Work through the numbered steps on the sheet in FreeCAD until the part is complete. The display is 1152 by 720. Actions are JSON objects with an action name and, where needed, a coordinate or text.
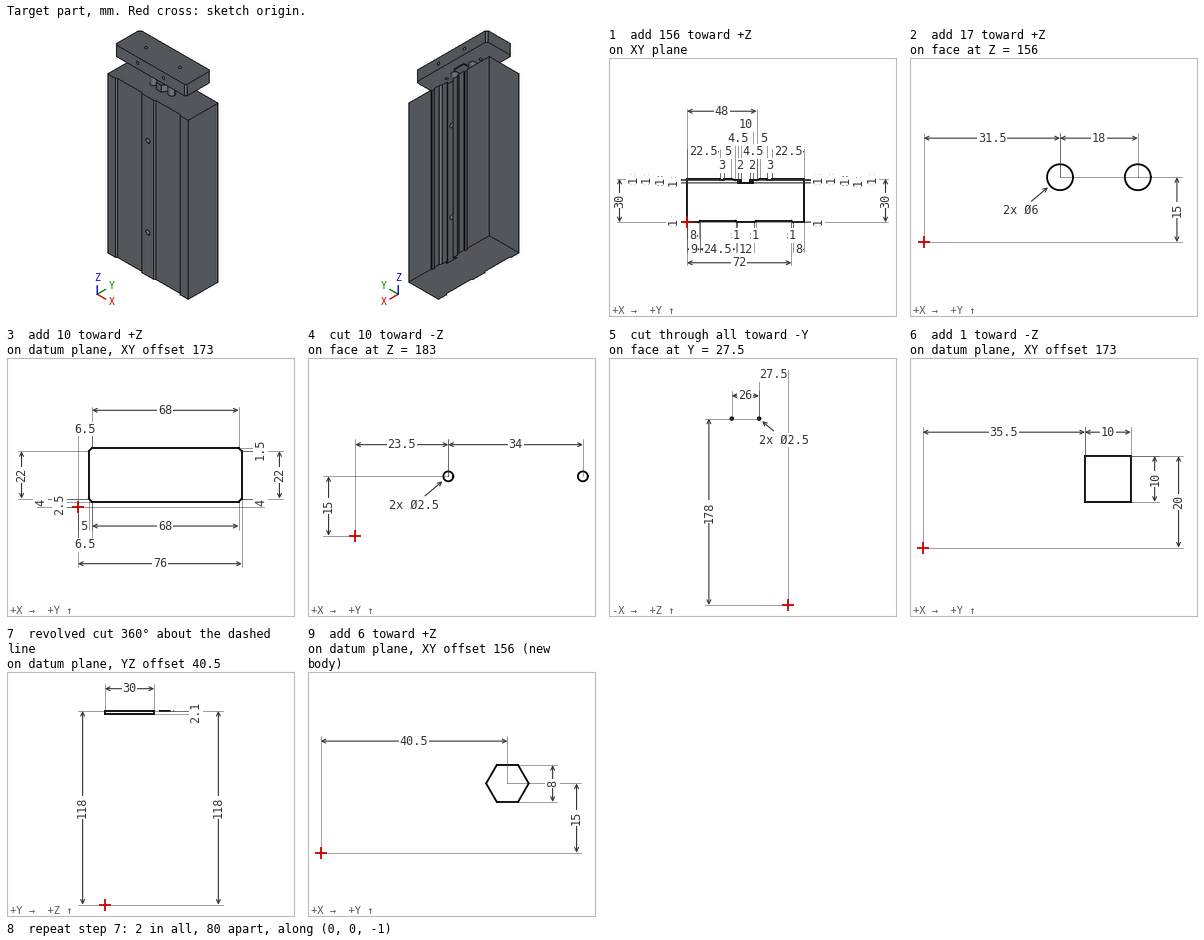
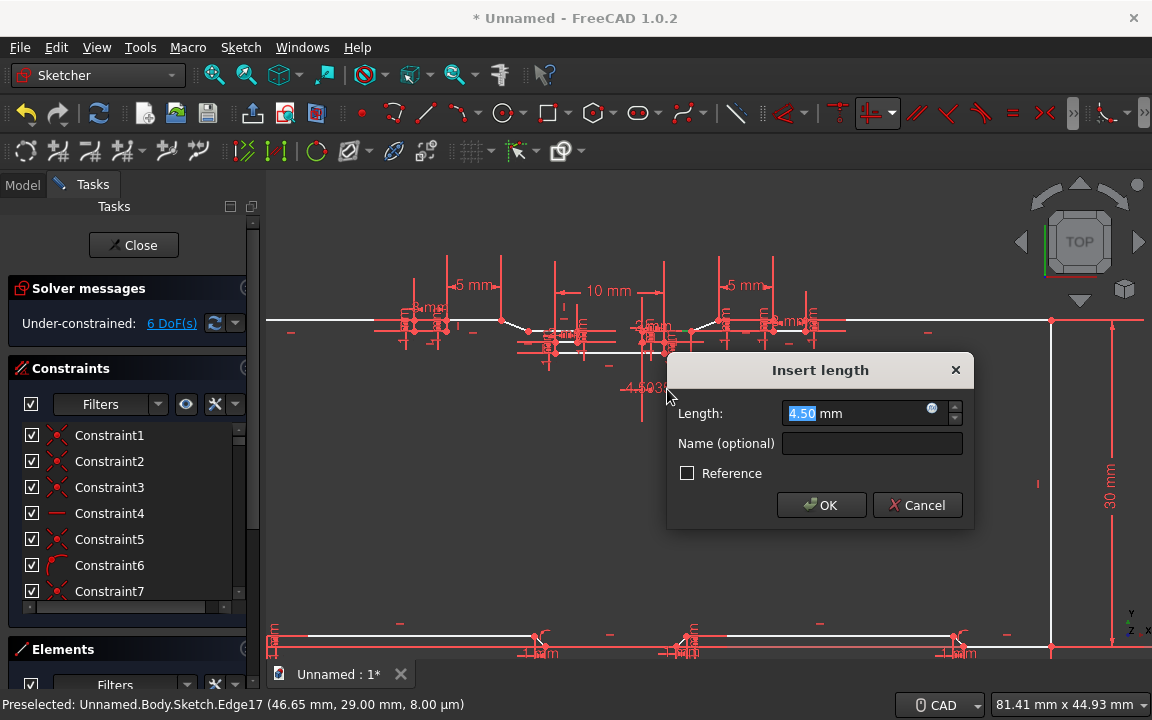
{"action": "type", "text": "4.5"}
{"action": "key", "text": "Return"}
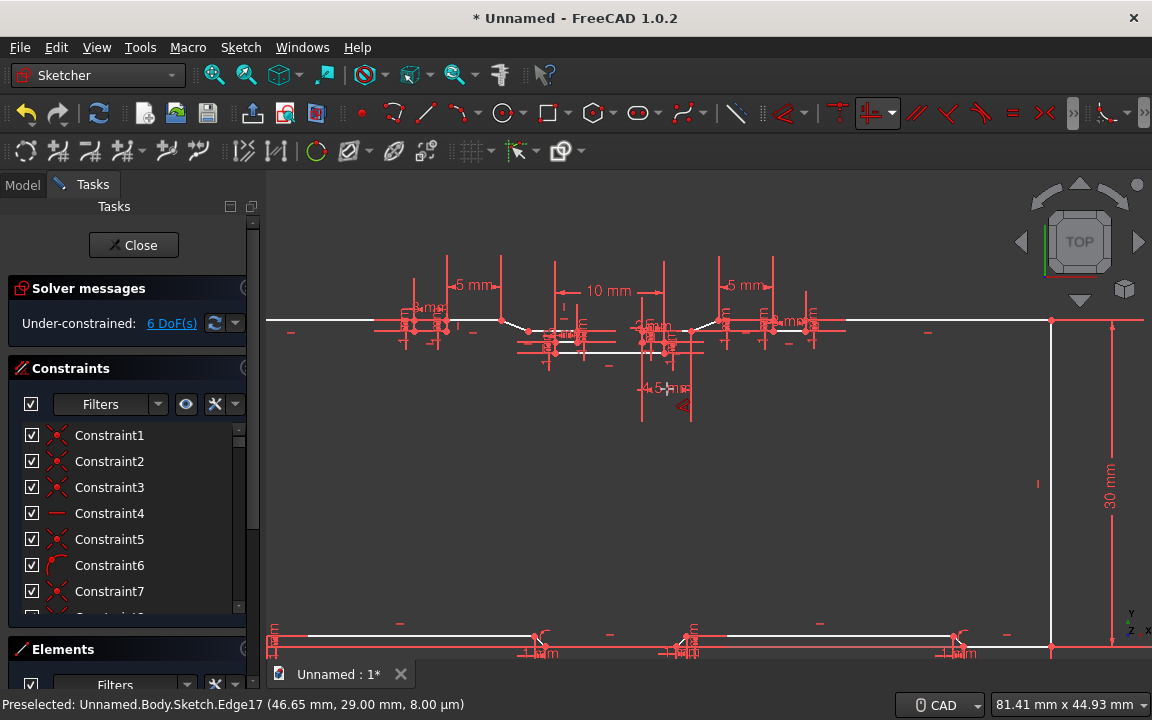
{"action": "scroll", "coordinate": [563, 331], "scroll_direction": "up", "scroll_amount": 2}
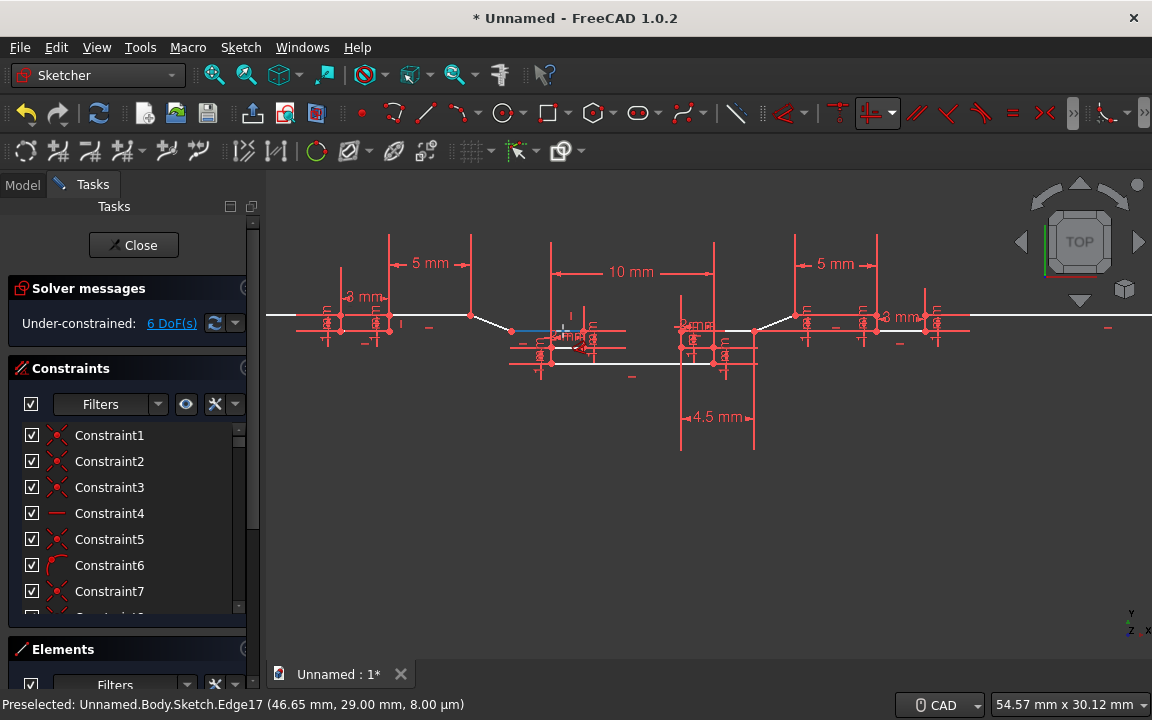
{"action": "left_click", "coordinate": [562, 331]}
{"action": "left_click", "coordinate": [548, 297]}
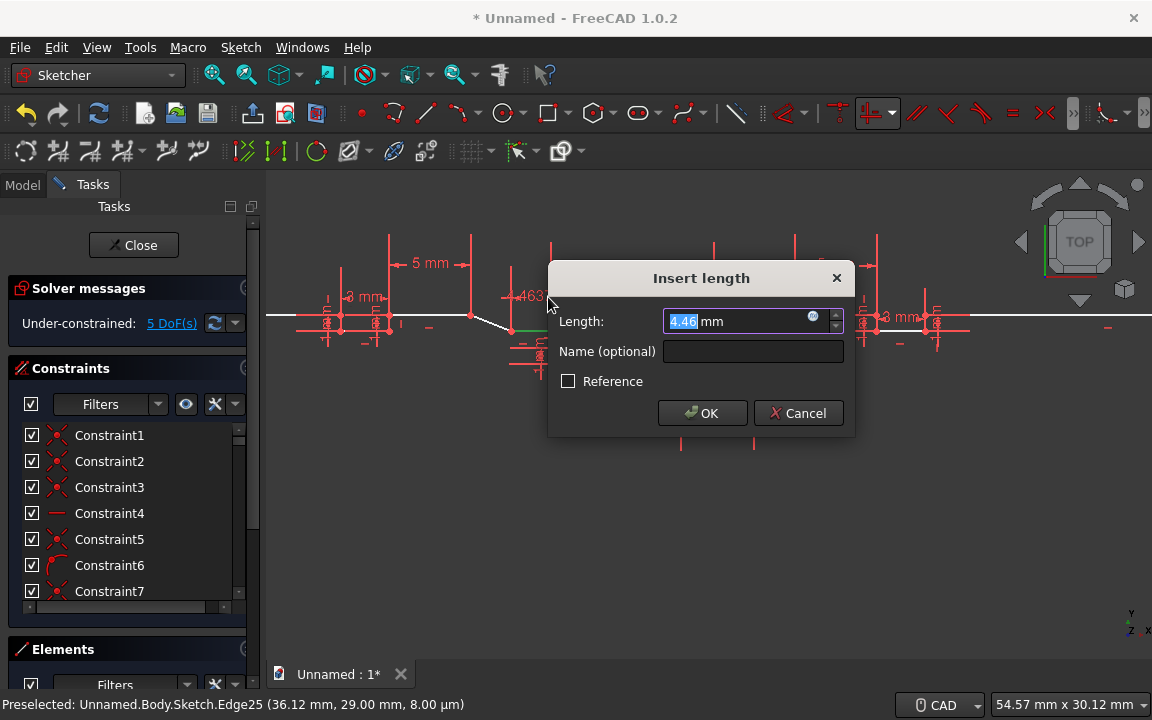
{"action": "type", "text": "4.5"}
{"action": "key", "text": "Return"}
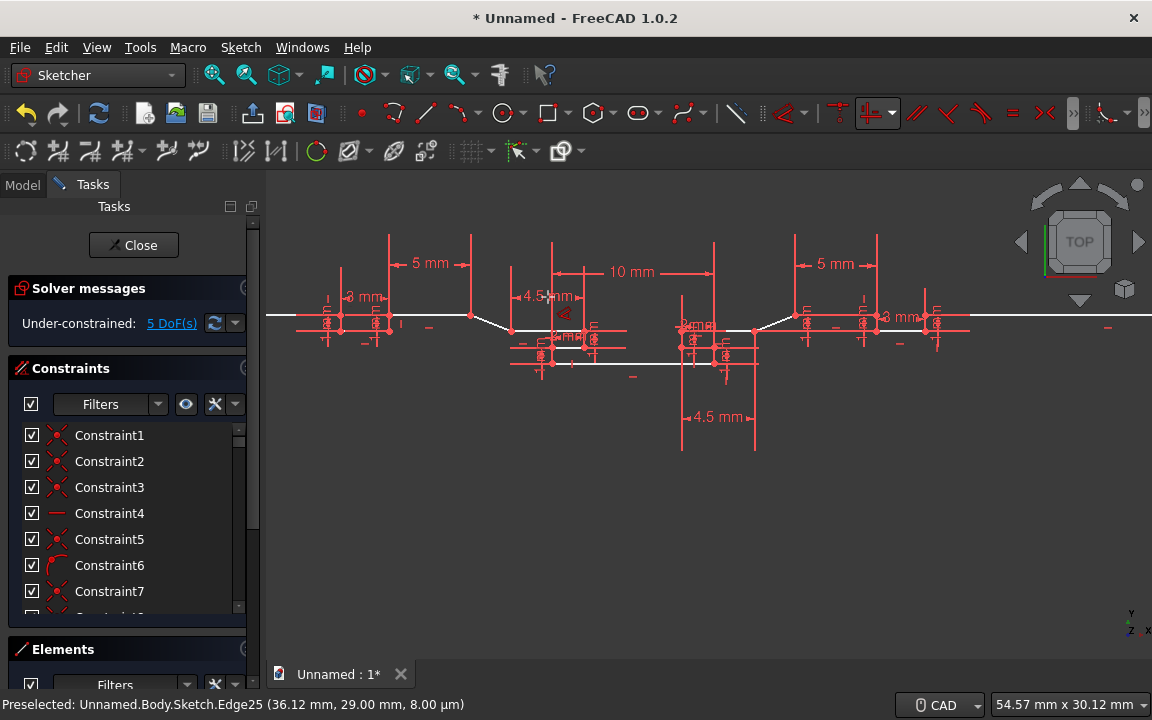
{"action": "scroll", "coordinate": [645, 331], "scroll_direction": "down", "scroll_amount": 5}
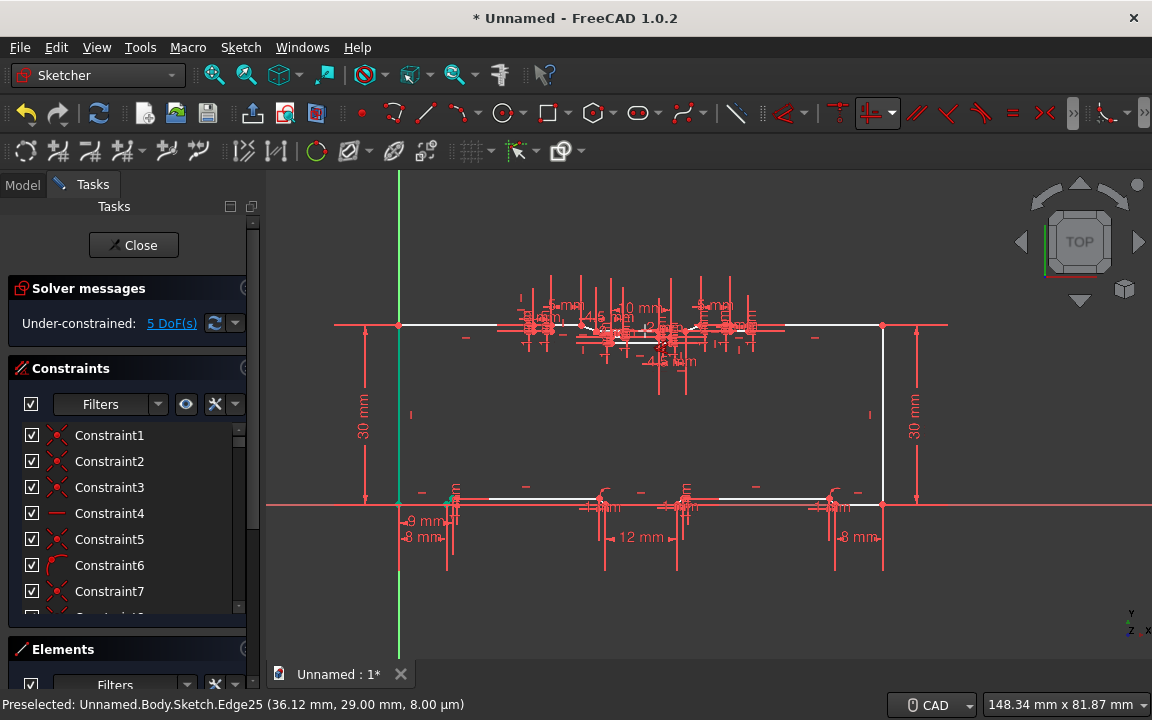
{"action": "scroll", "coordinate": [829, 499], "scroll_direction": "up", "scroll_amount": 2}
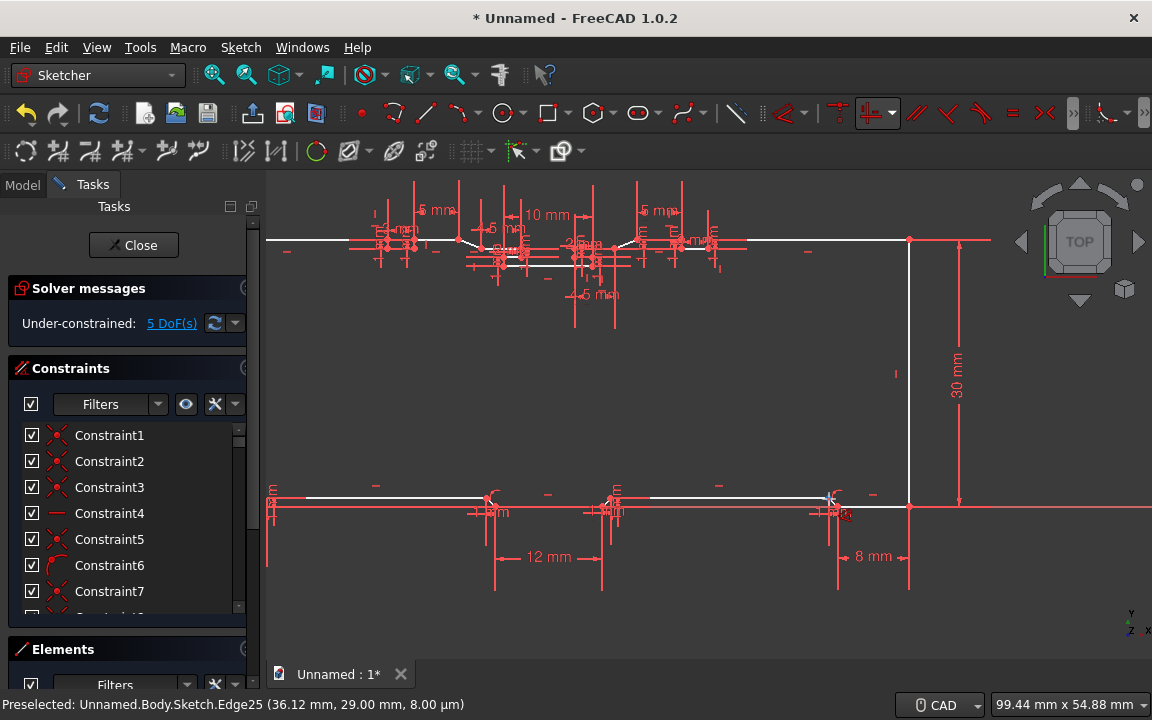
{"action": "left_click", "coordinate": [829, 498]}
{"action": "left_click", "coordinate": [438, 541]}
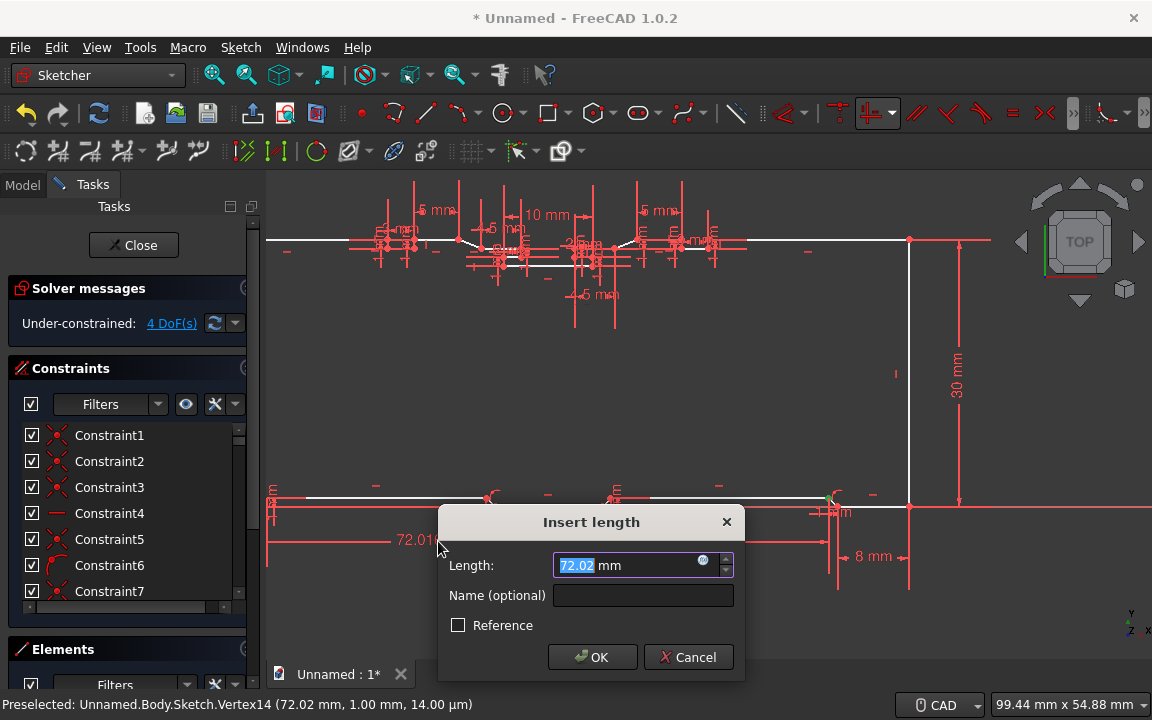
{"action": "type", "text": "72"}
{"action": "key", "text": "Return"}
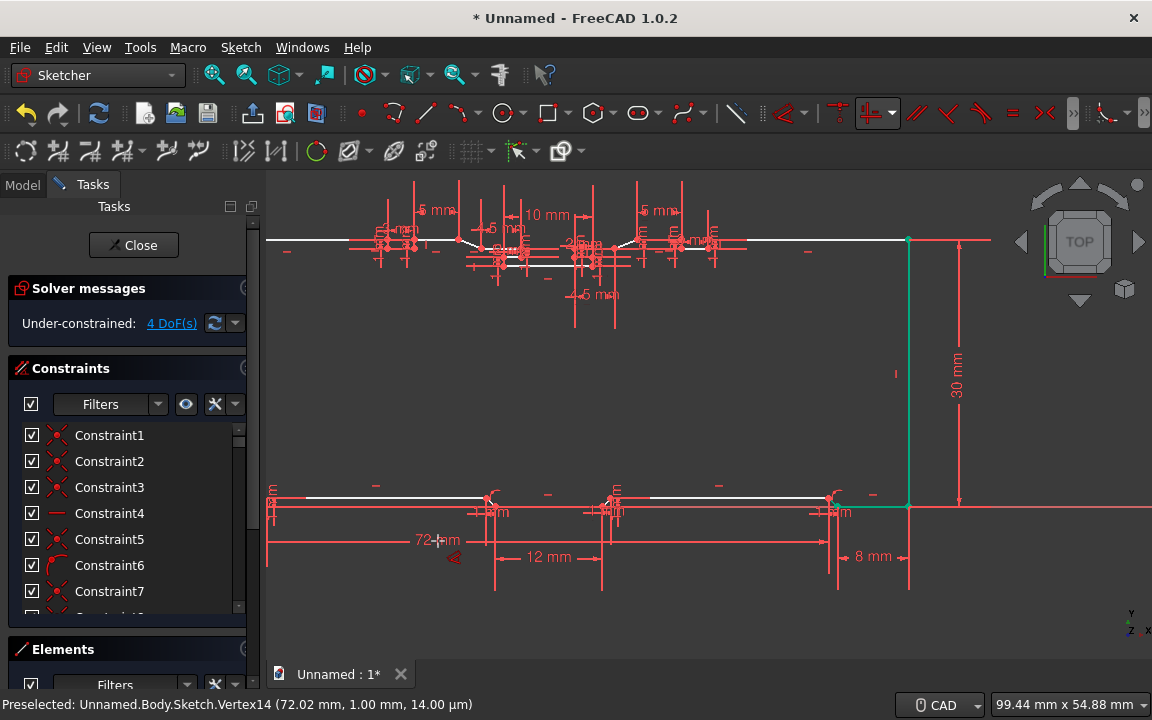
{"action": "left_click", "coordinate": [615, 249]}
{"action": "left_click", "coordinate": [342, 541]}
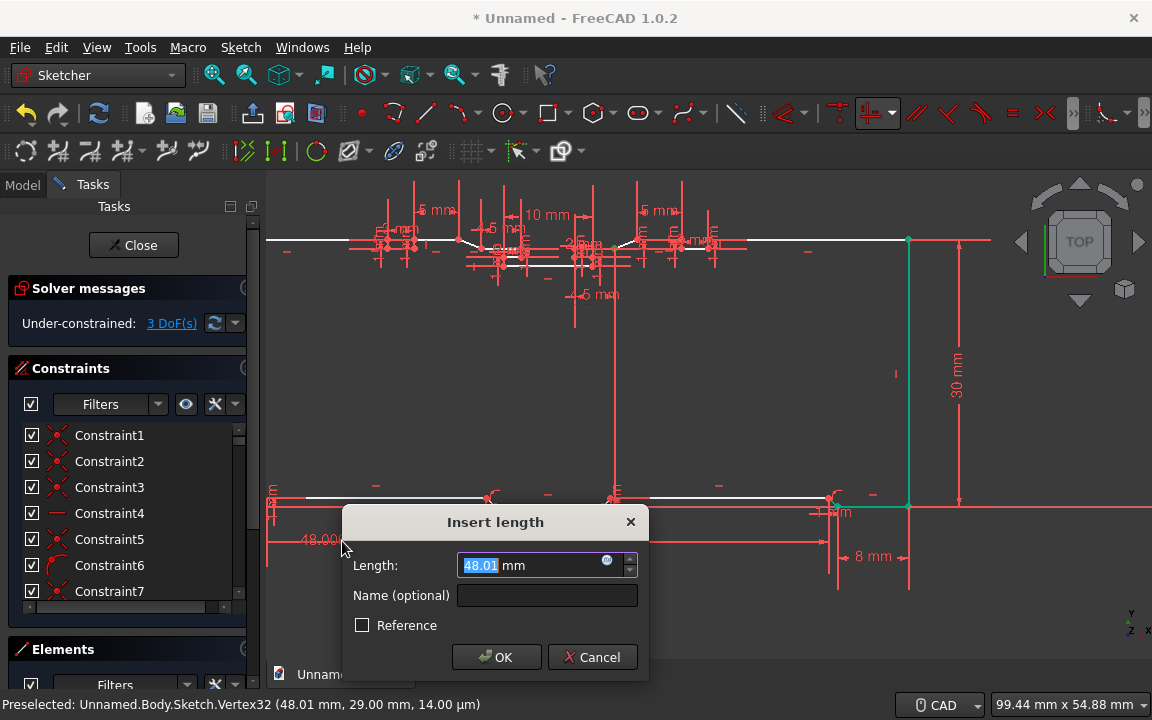
{"action": "type", "text": "48"}
{"action": "key", "text": "Return"}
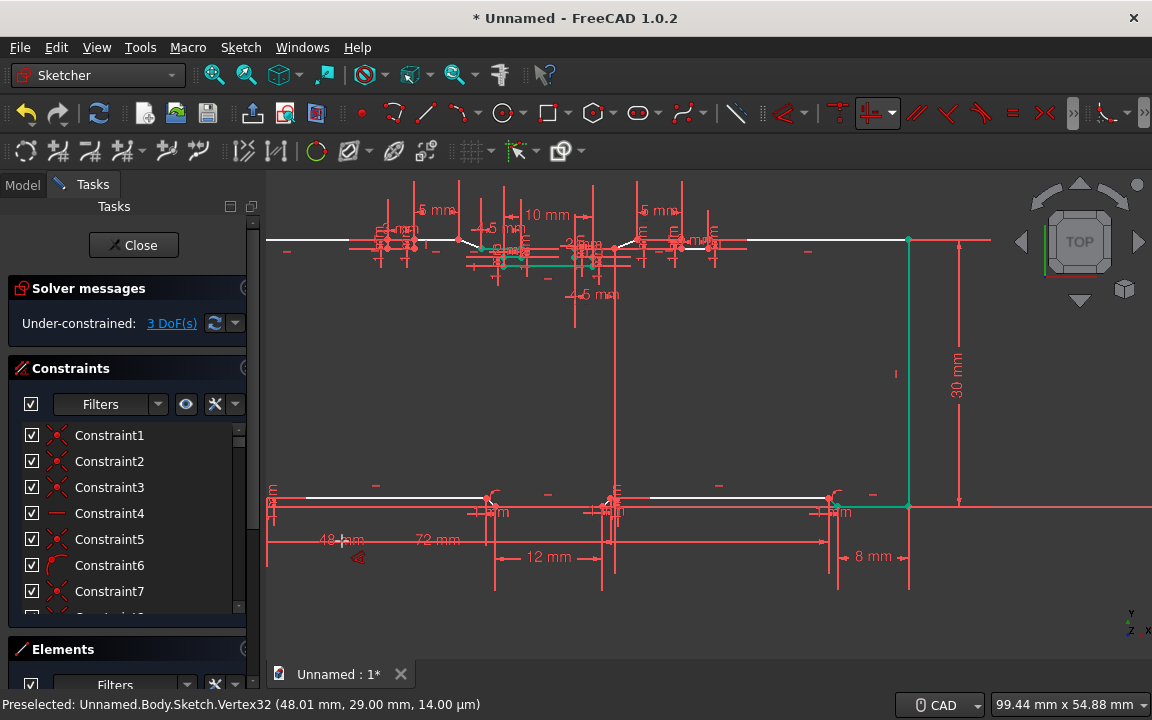
{"action": "scroll", "coordinate": [333, 498], "scroll_direction": "up", "scroll_amount": 3}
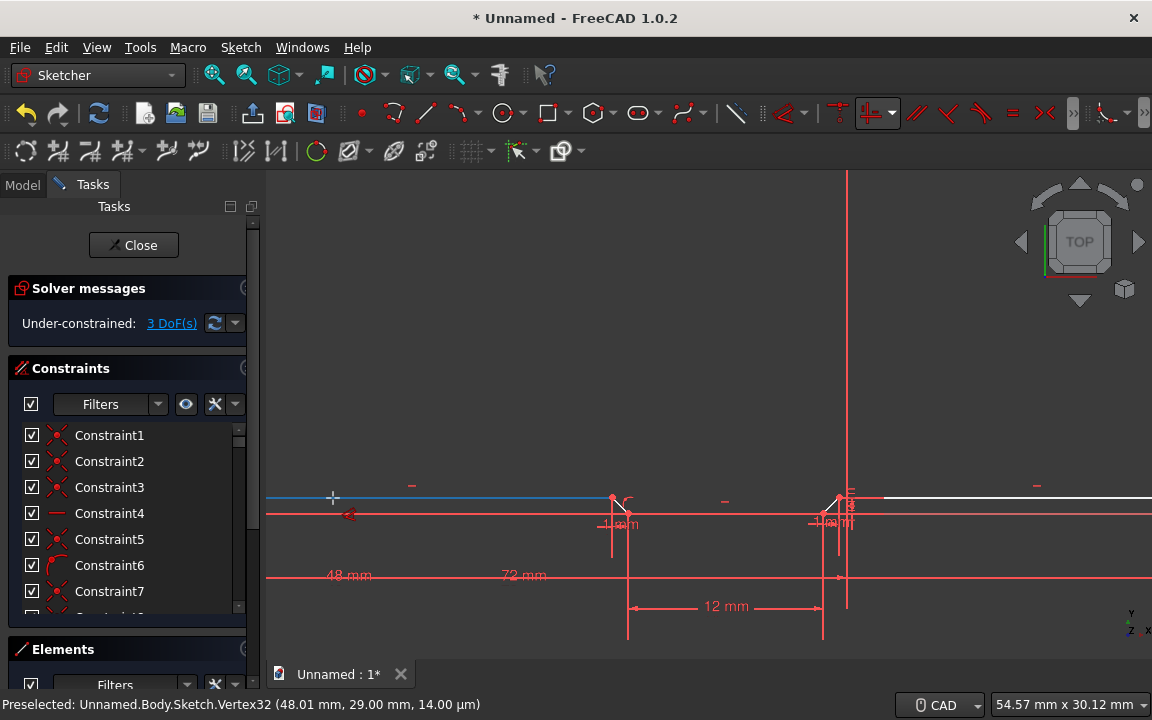
{"action": "left_click", "coordinate": [333, 498]}
{"action": "left_click", "coordinate": [453, 532]}